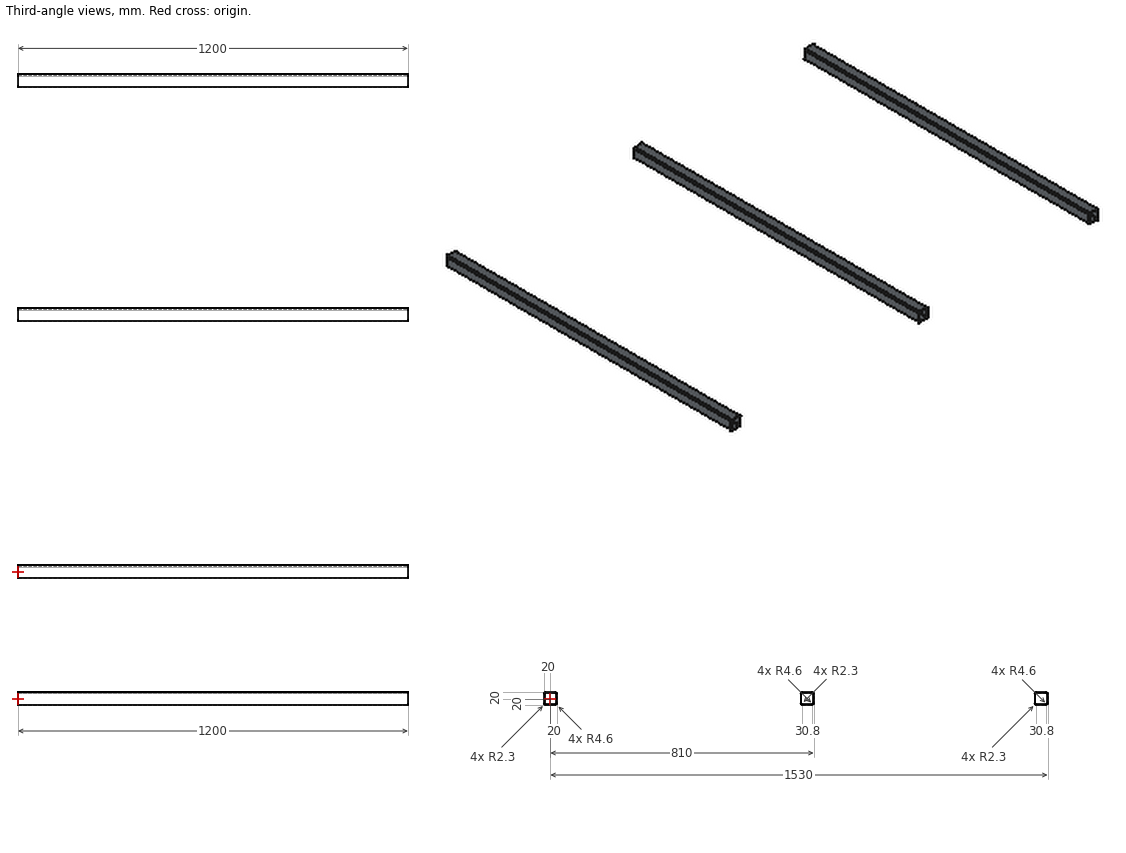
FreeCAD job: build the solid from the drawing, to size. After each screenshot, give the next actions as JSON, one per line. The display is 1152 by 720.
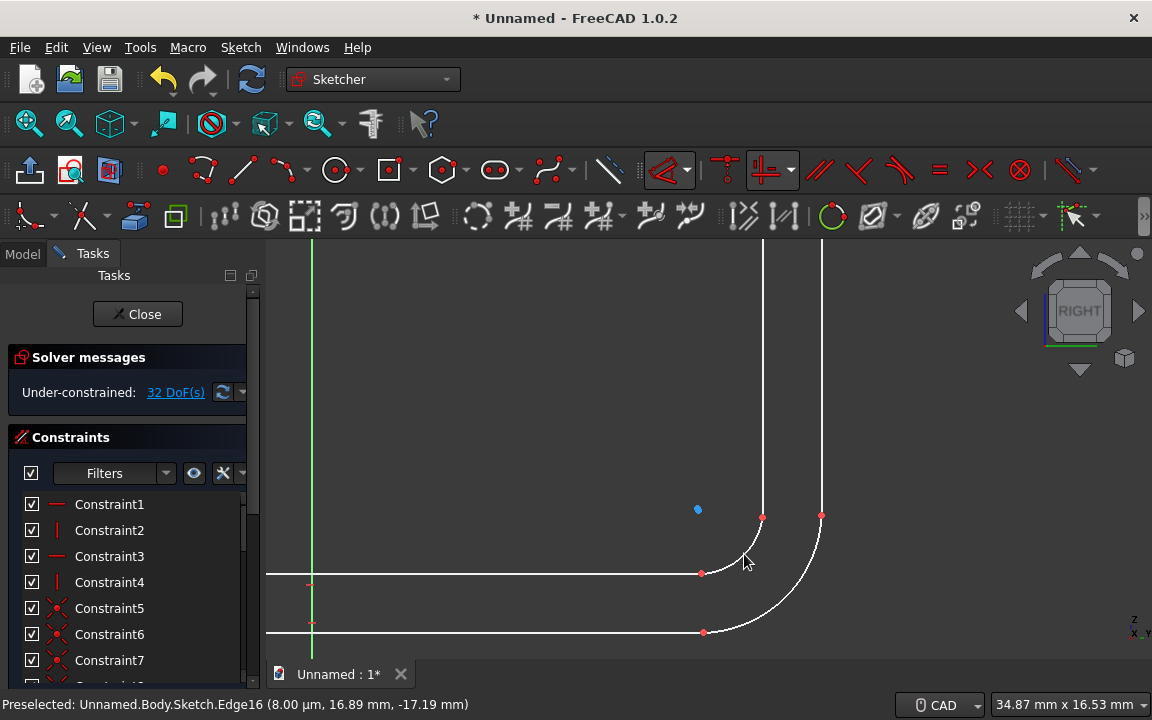
{"action": "scroll", "coordinate": [748, 556], "scroll_direction": "down", "scroll_amount": 7}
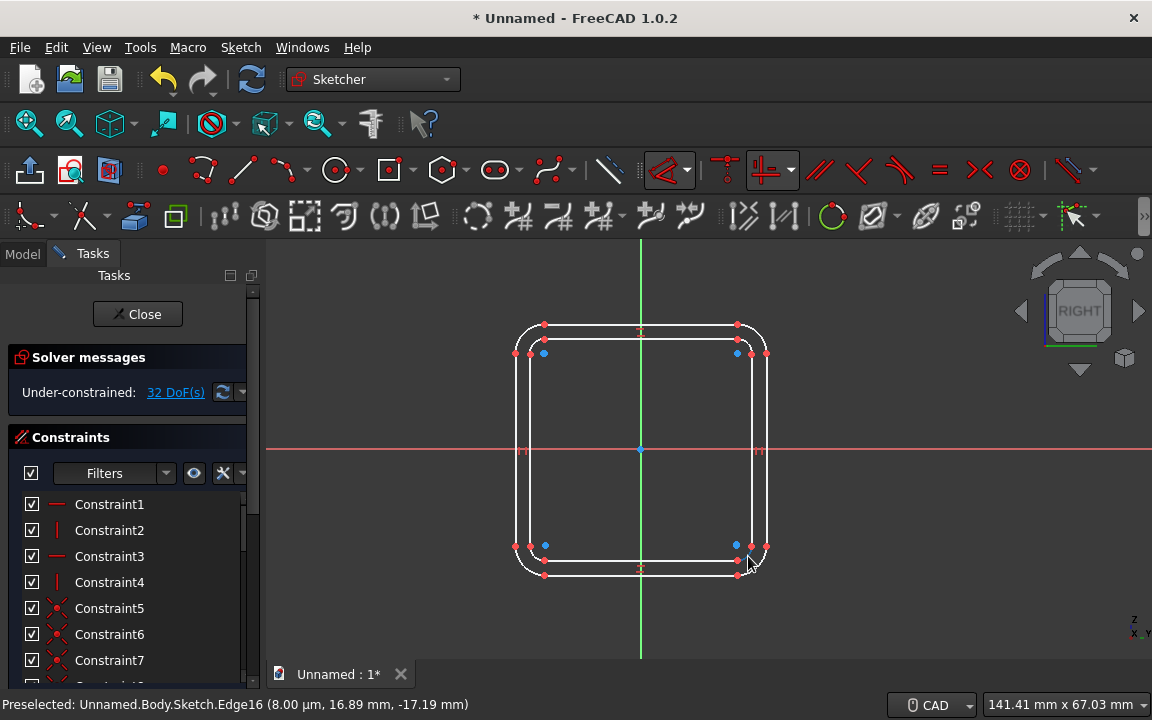
{"action": "left_click", "coordinate": [602, 576]}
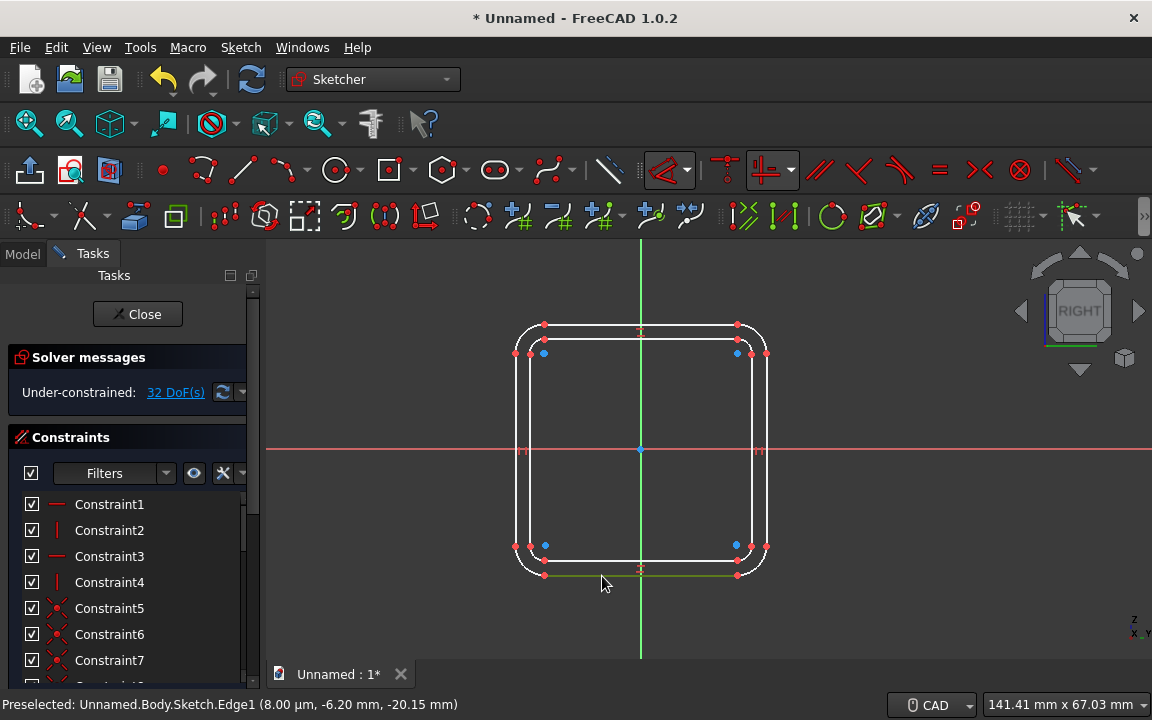
{"action": "left_click", "coordinate": [750, 572]}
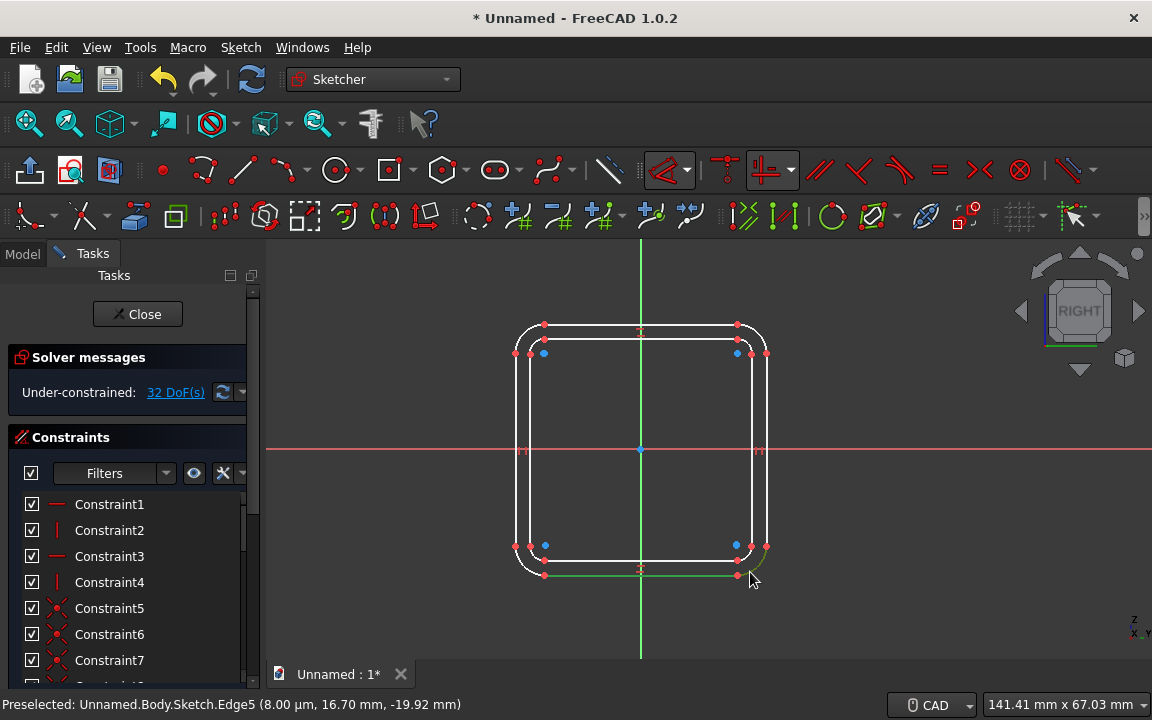
{"action": "key", "text": "t"}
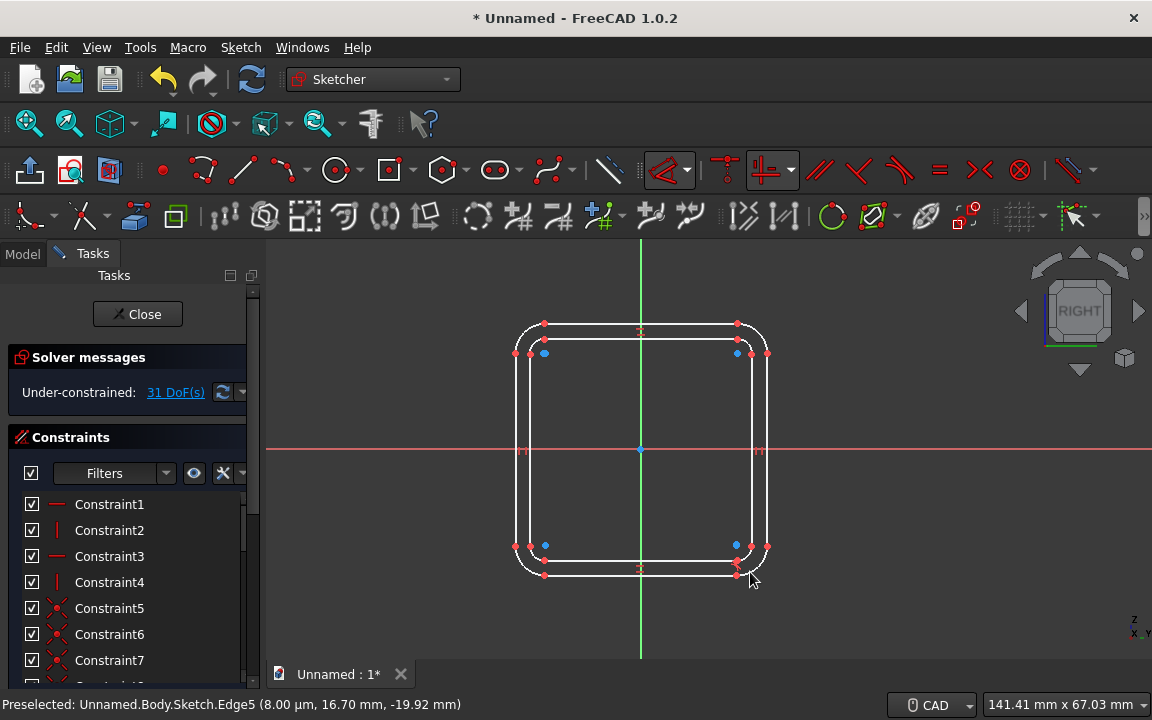
{"action": "left_click", "coordinate": [602, 576]}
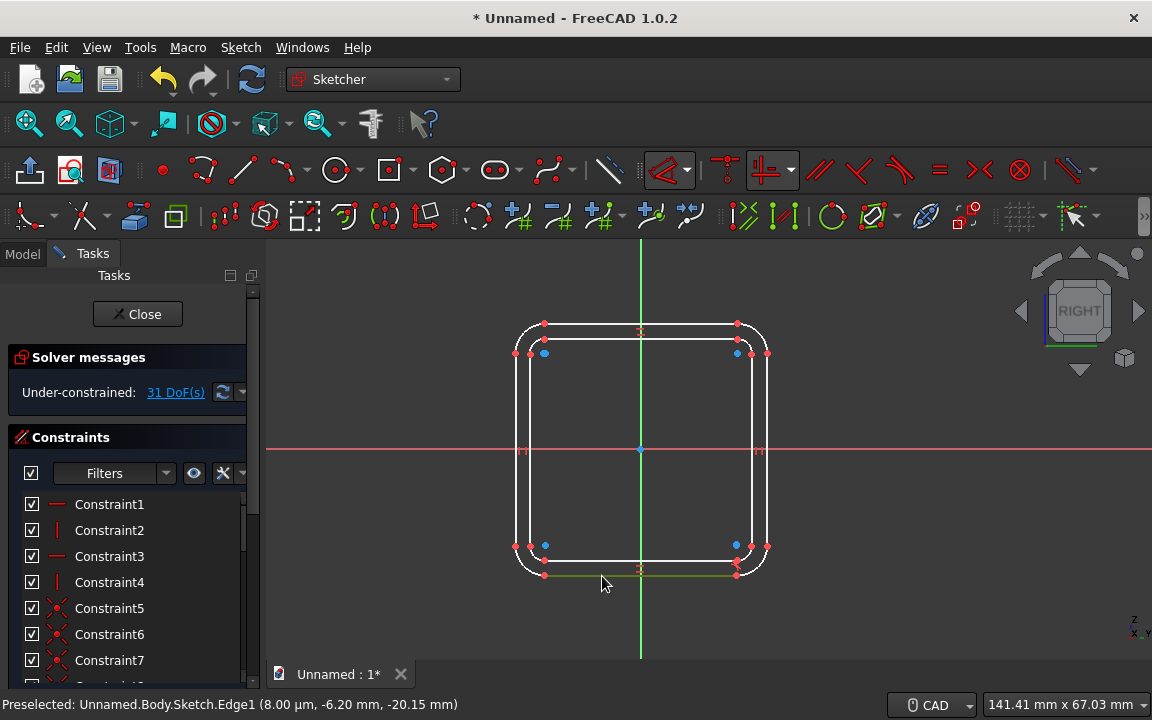
{"action": "left_click", "coordinate": [519, 559]}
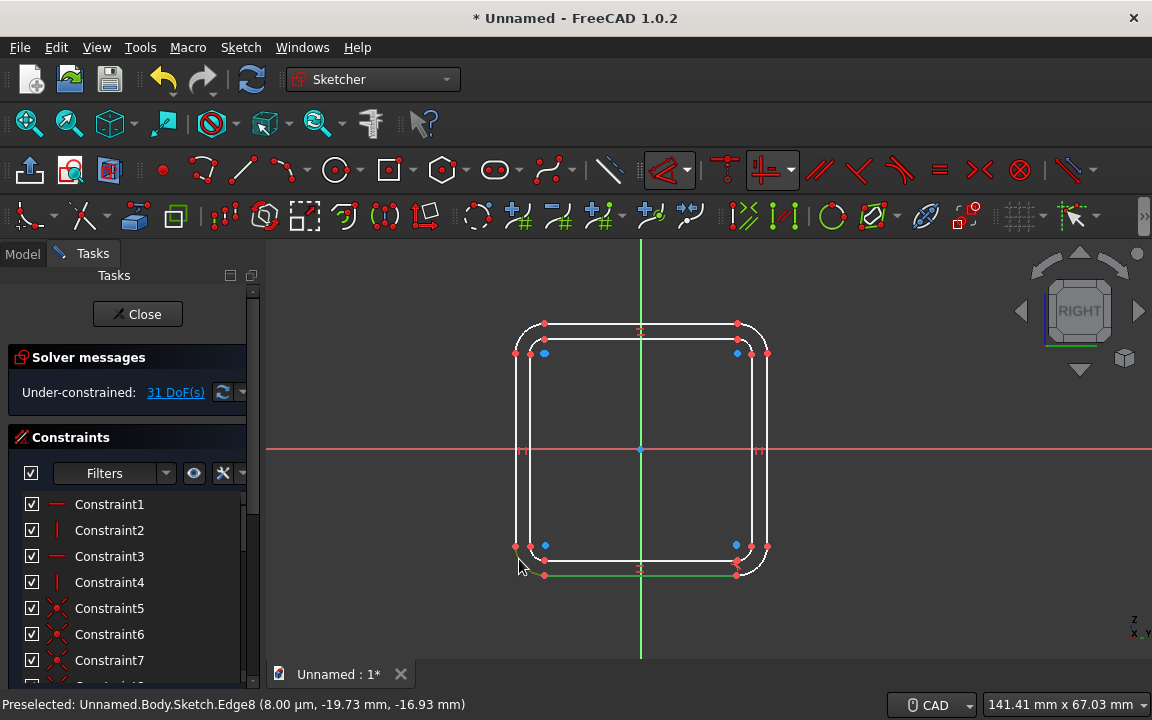
{"action": "key", "text": "t"}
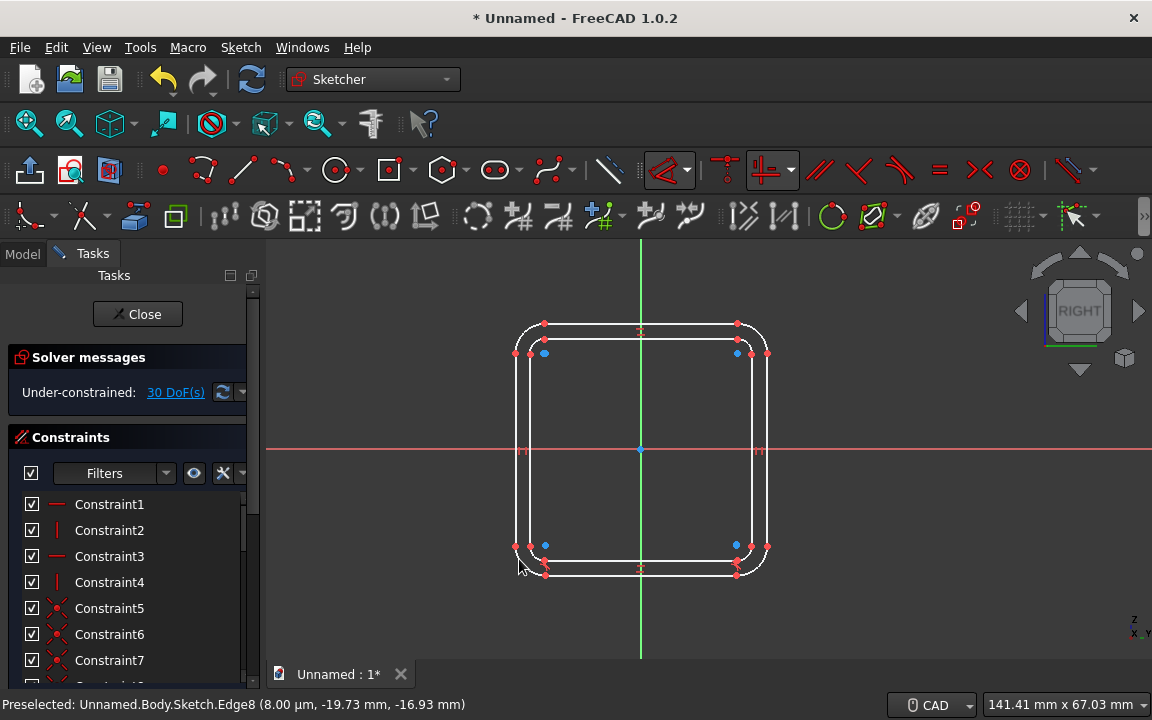
{"action": "left_click", "coordinate": [767, 489]}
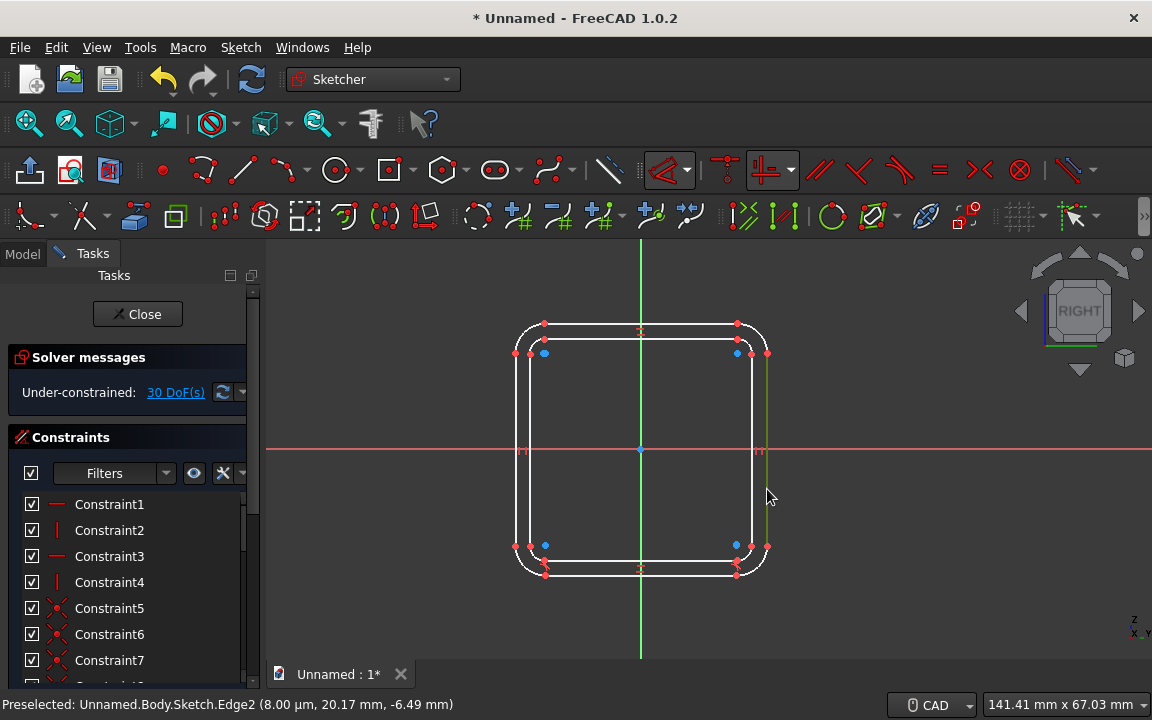
{"action": "left_click", "coordinate": [750, 572]}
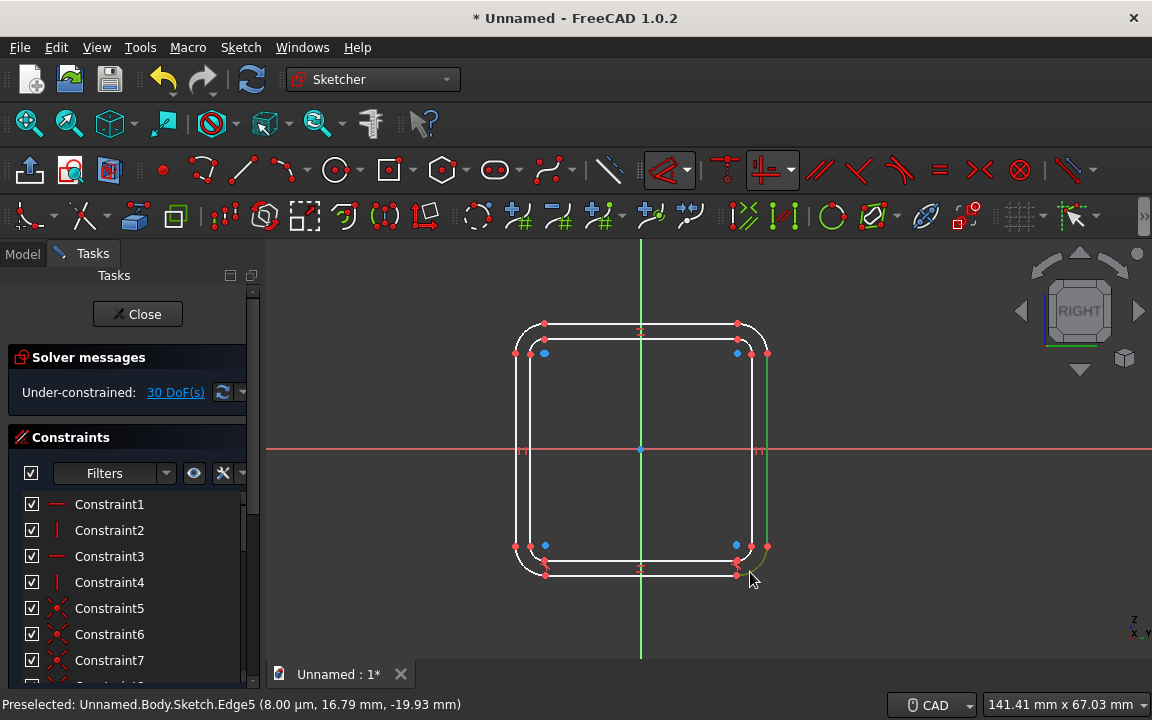
{"action": "key", "text": "t"}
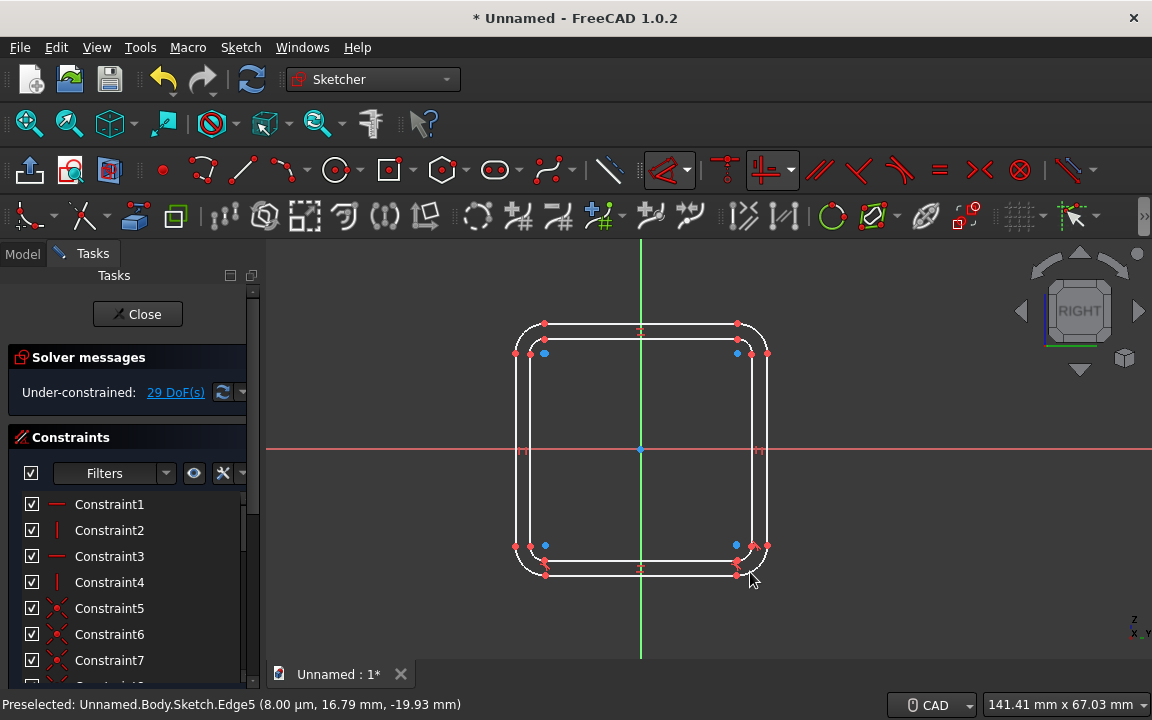
{"action": "left_click", "coordinate": [767, 488]}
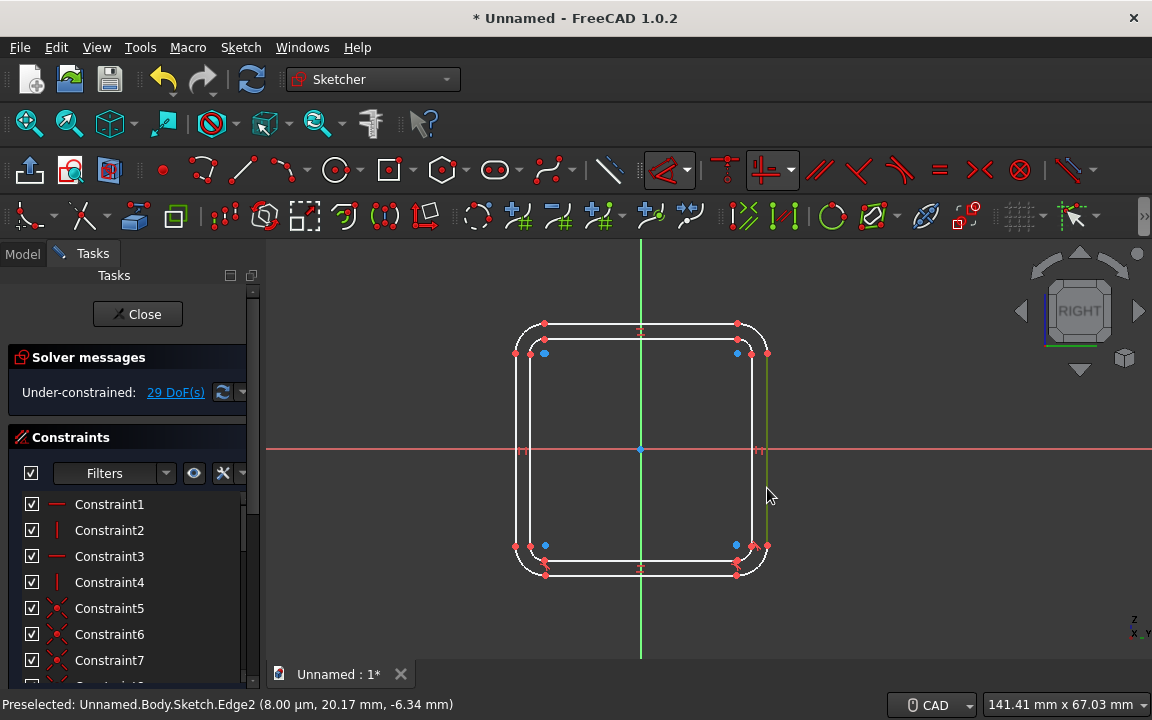
{"action": "left_click", "coordinate": [764, 340]}